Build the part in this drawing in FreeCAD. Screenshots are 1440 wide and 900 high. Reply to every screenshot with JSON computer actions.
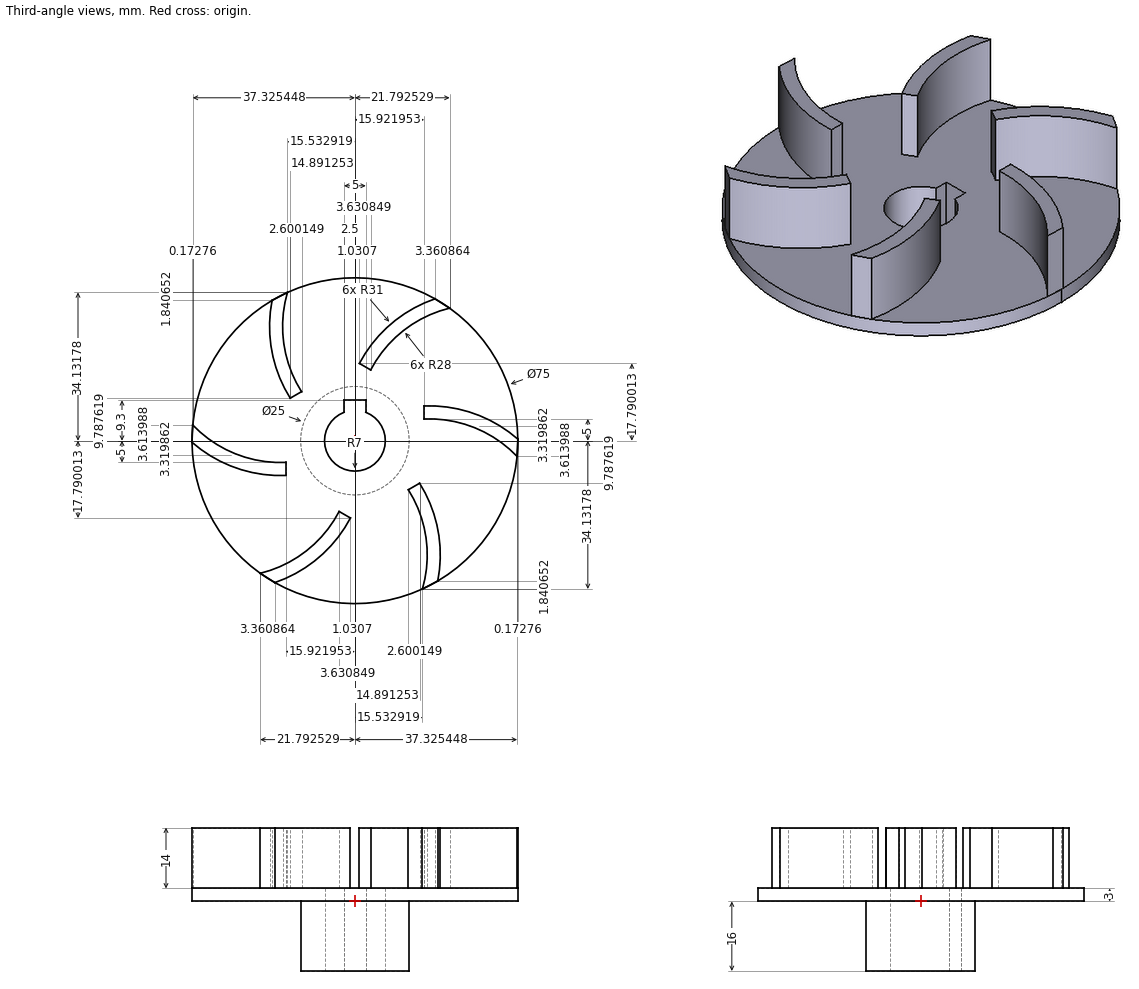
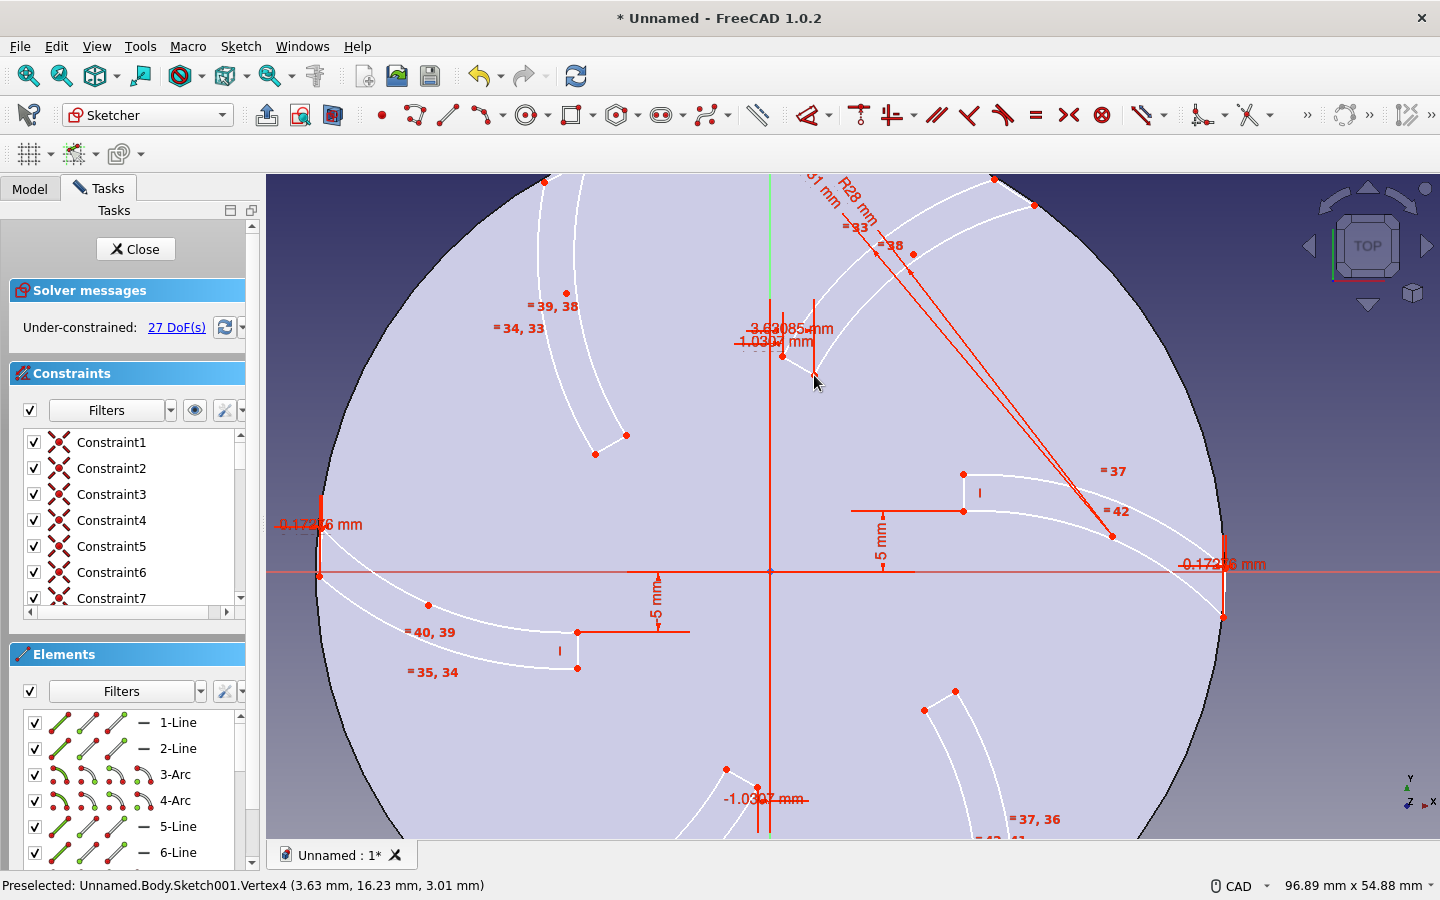
{"action": "scroll", "coordinate": [802, 427], "scroll_direction": "down", "scroll_amount": 3}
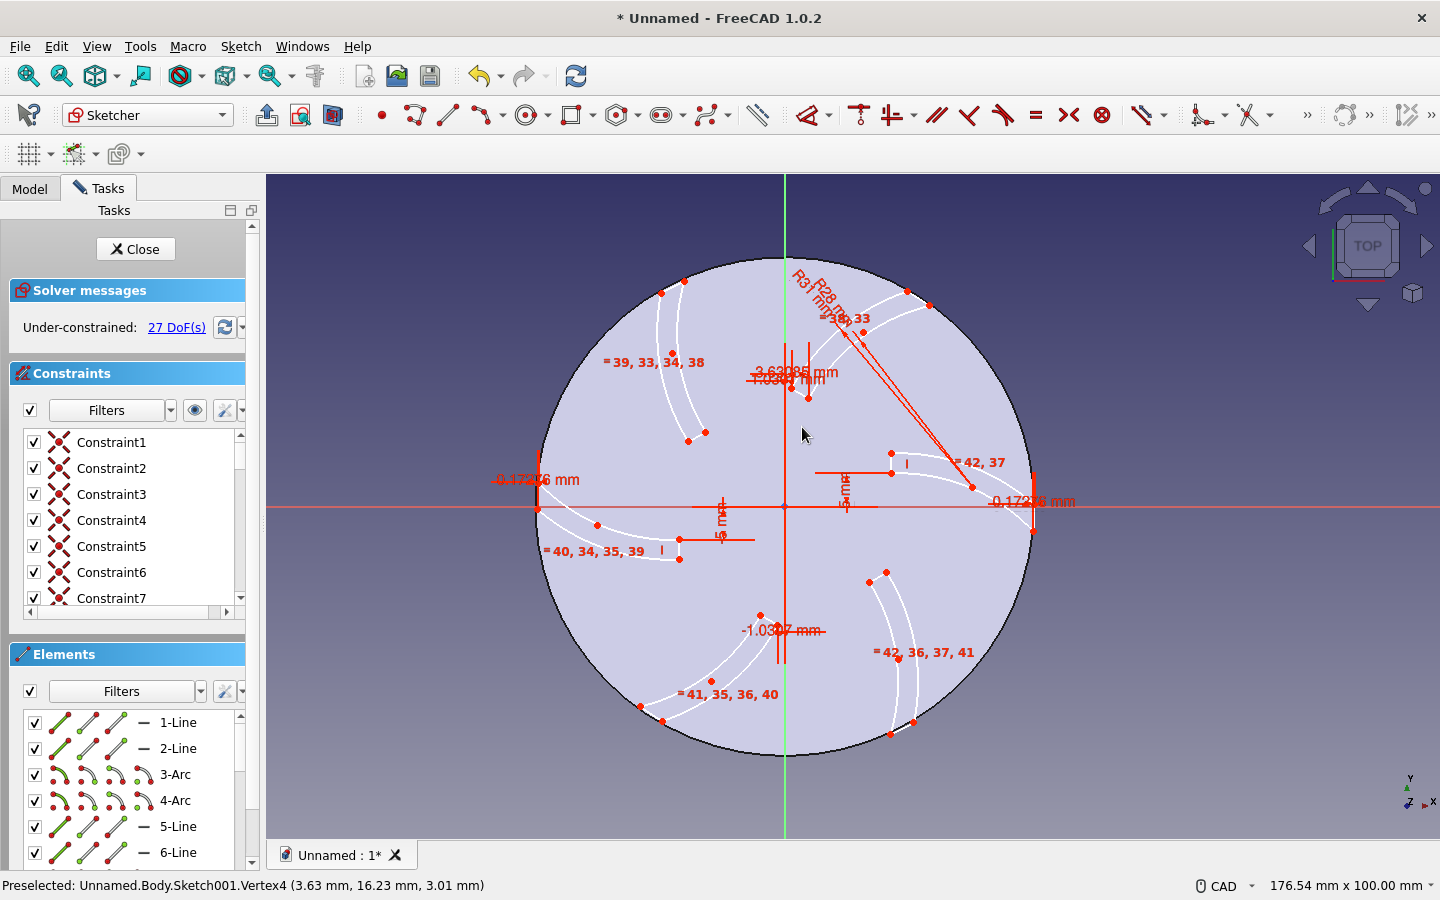
{"action": "left_click", "coordinate": [684, 281]}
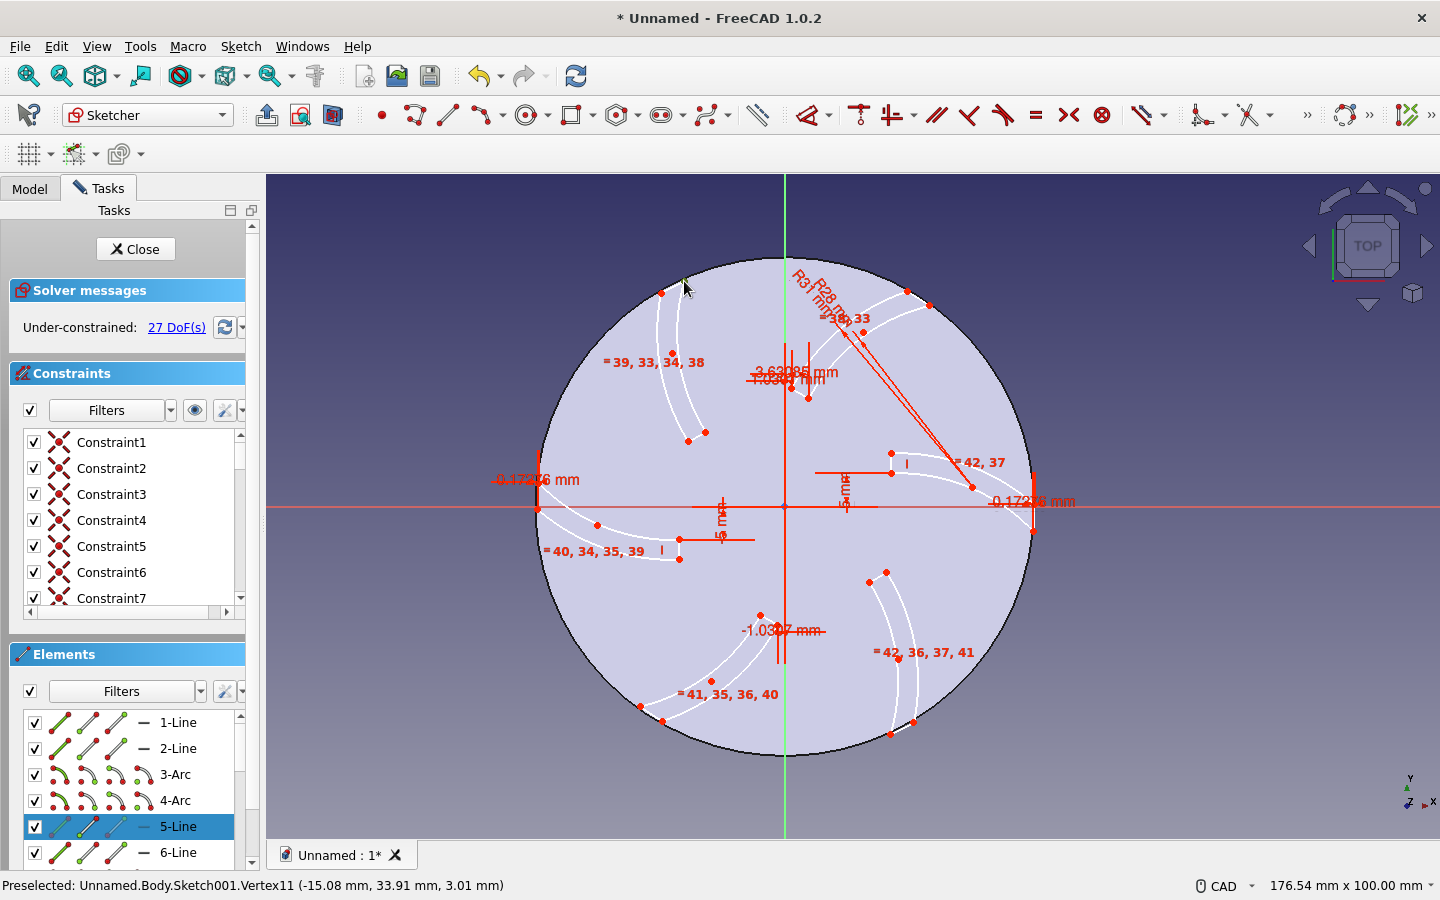
{"action": "key", "text": "i"}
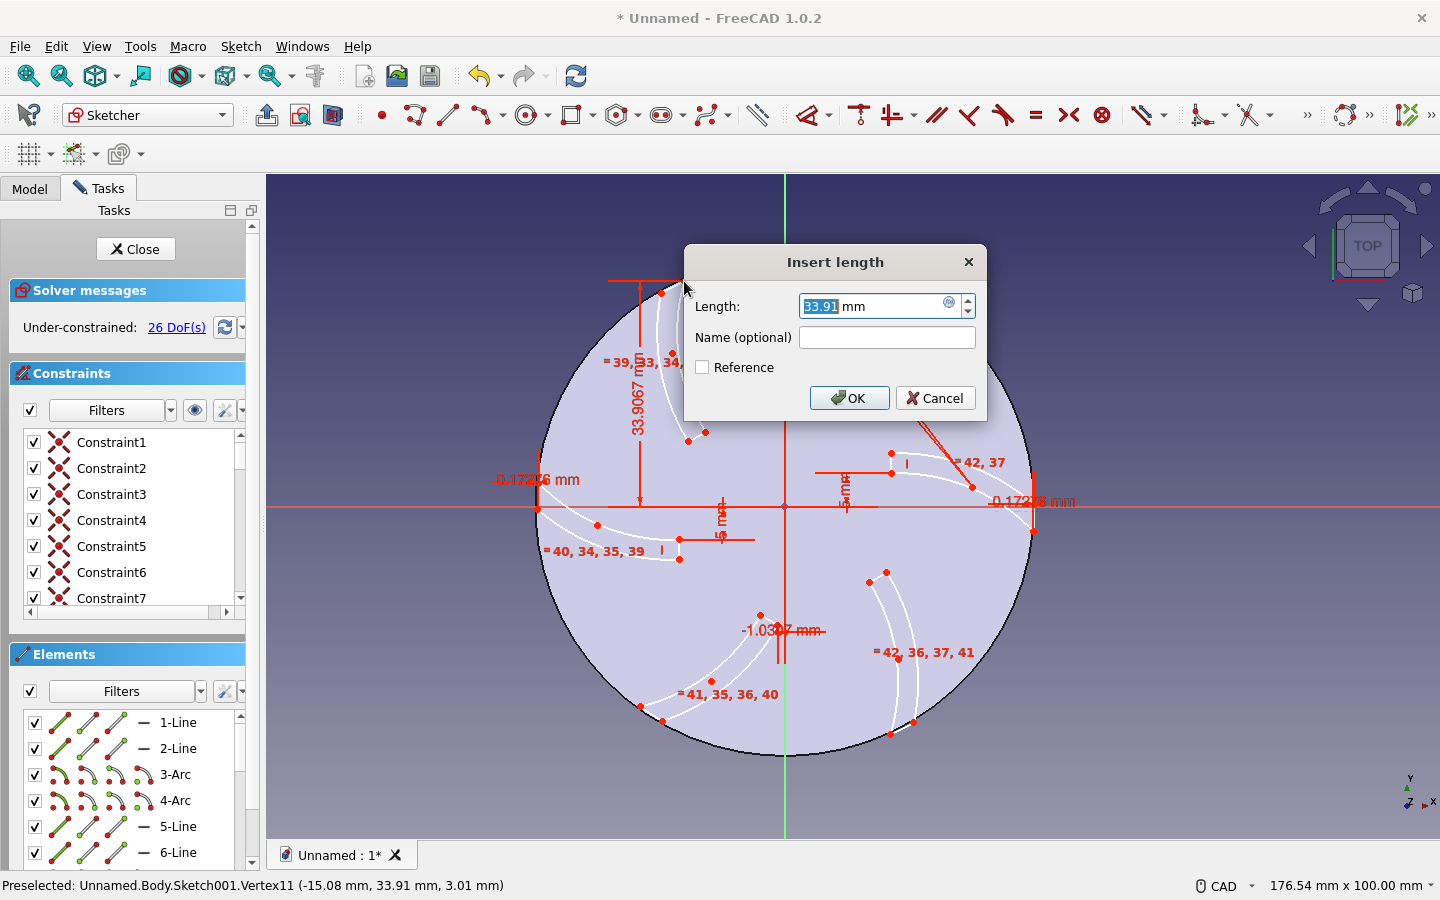
{"action": "type", "text": "34.13178"}
{"action": "key", "text": "Return"}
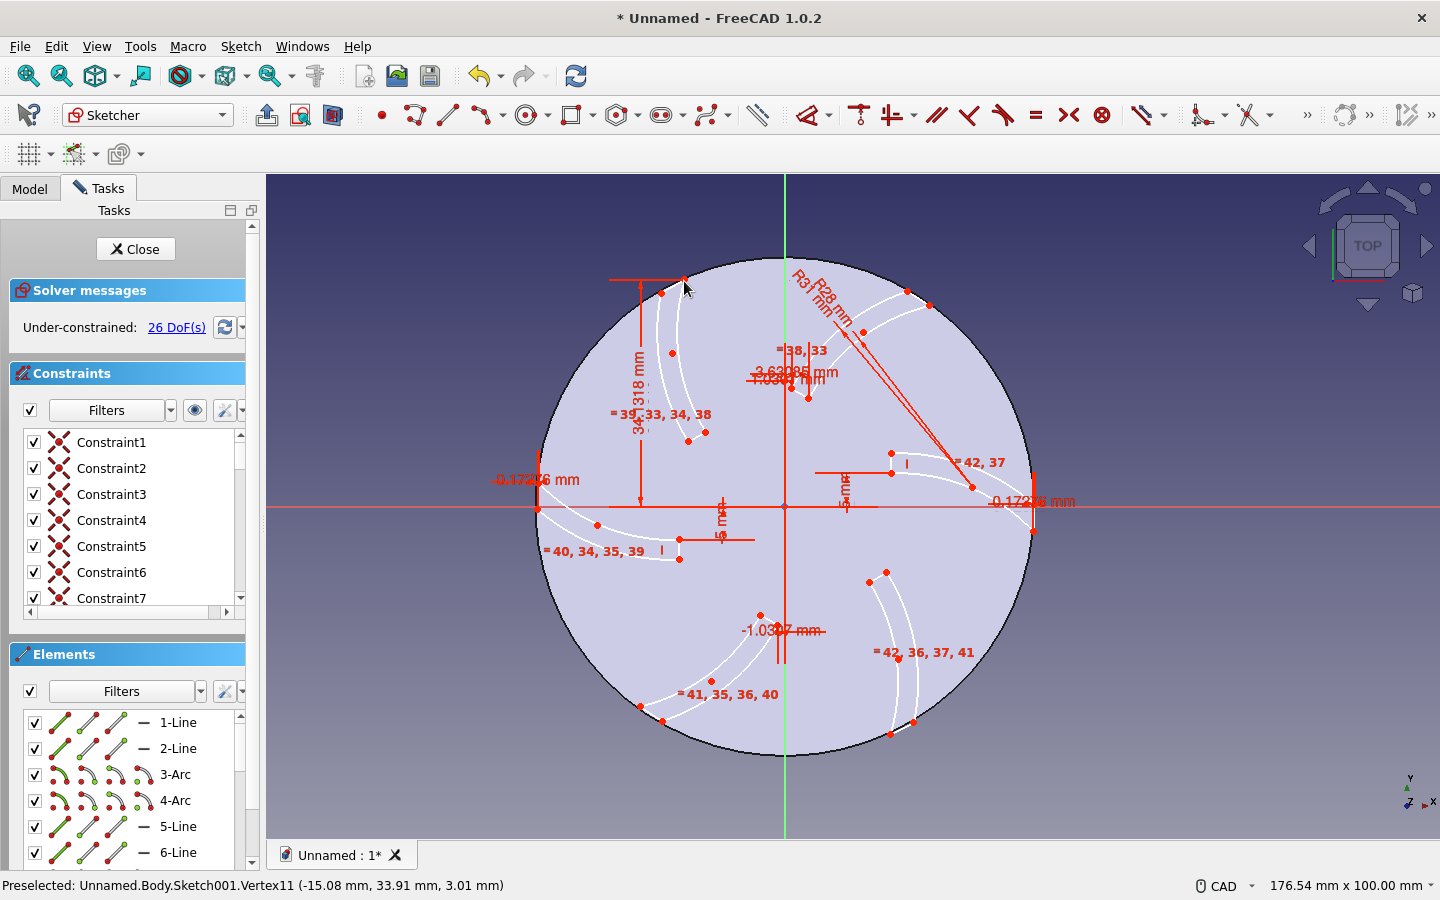
{"action": "left_click", "coordinate": [689, 442]}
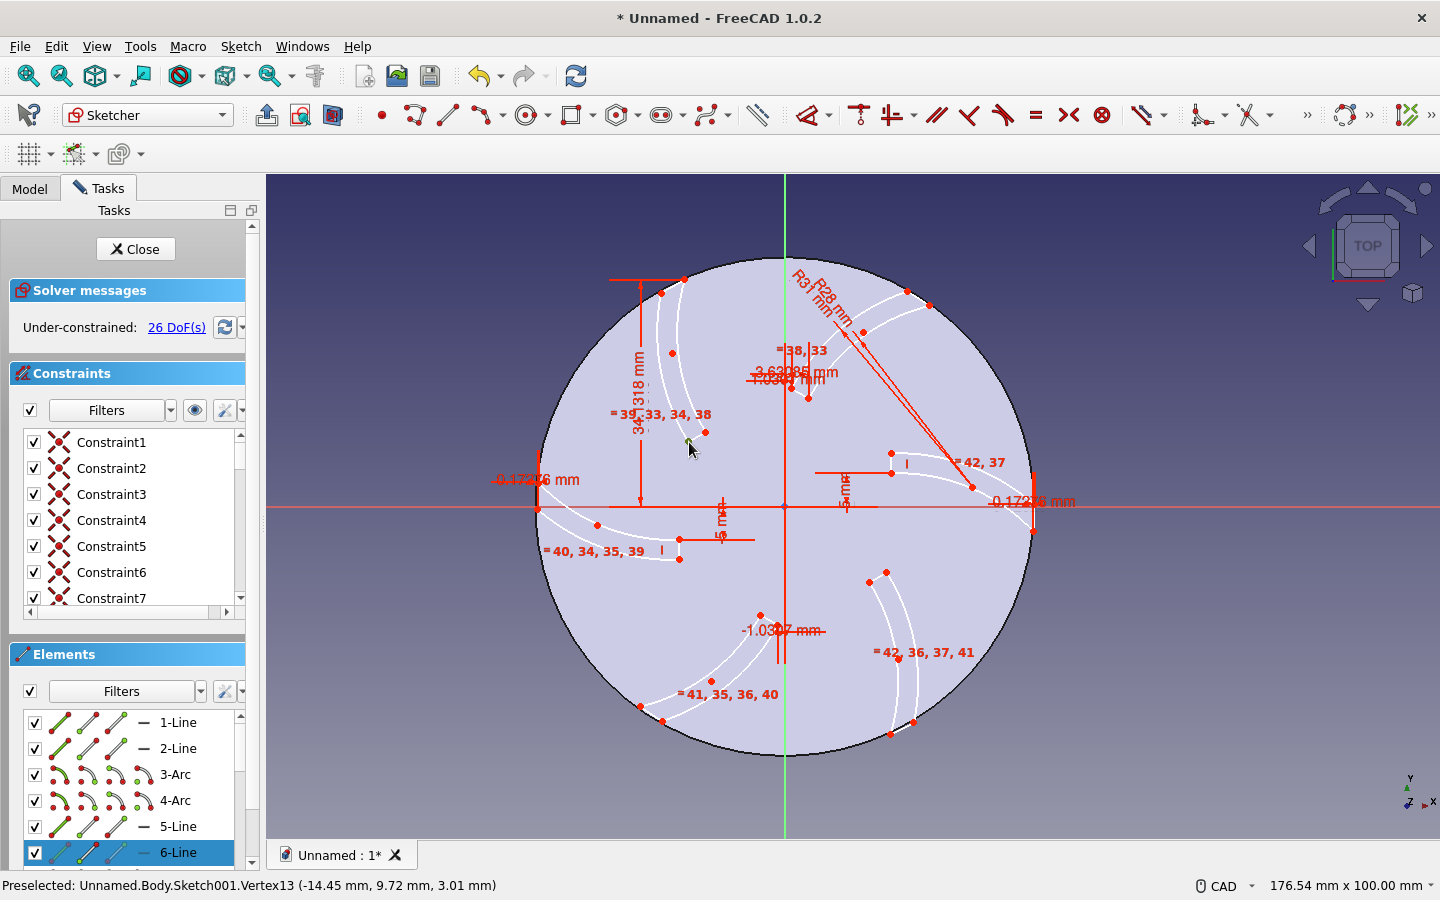
{"action": "key", "text": "i"}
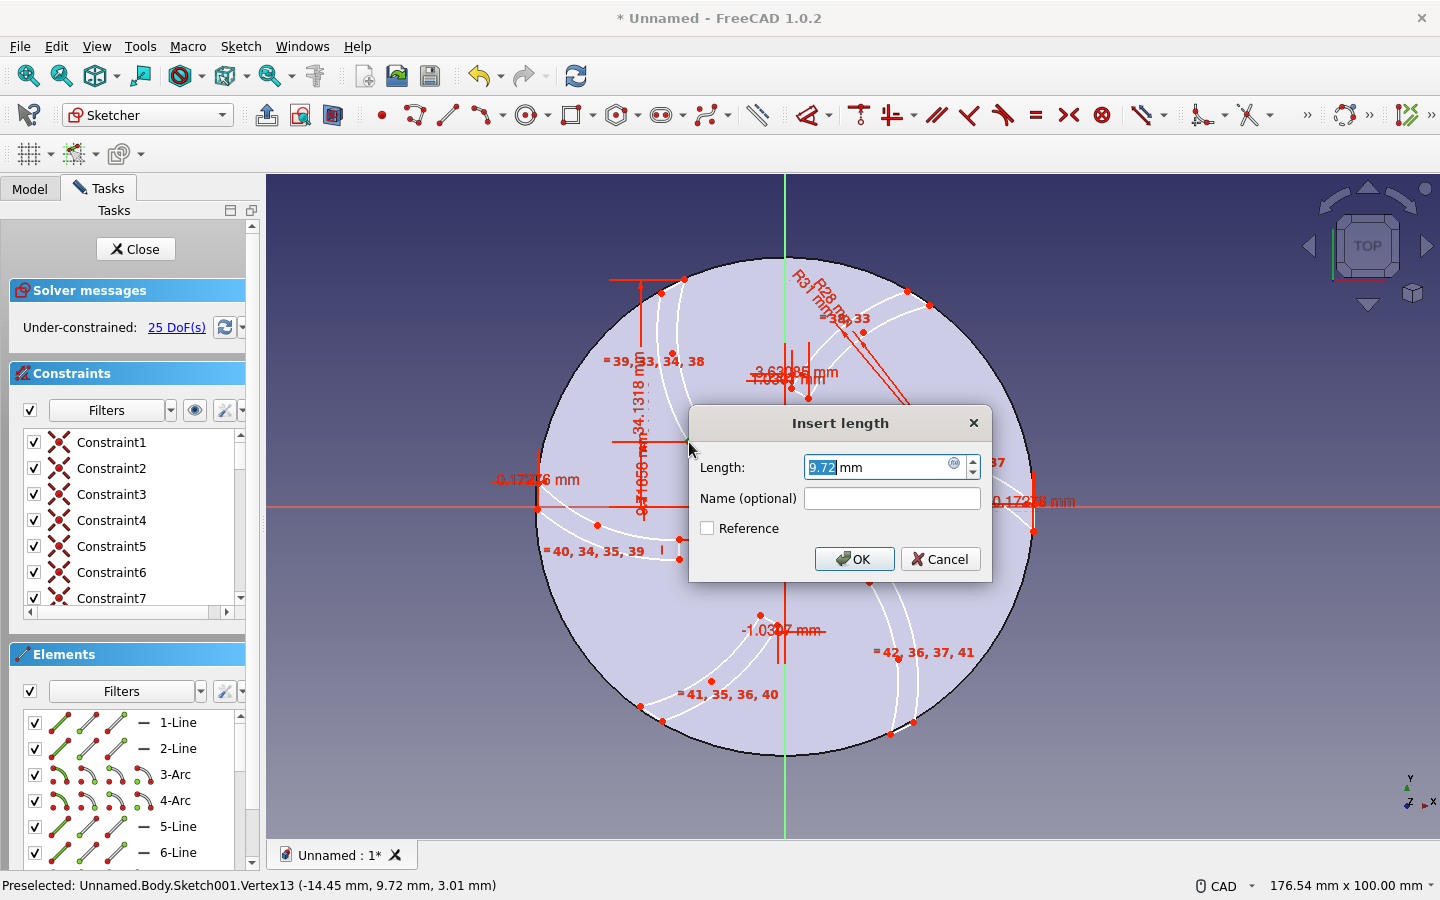
{"action": "type", "text": "9.787619"}
{"action": "key", "text": "Return"}